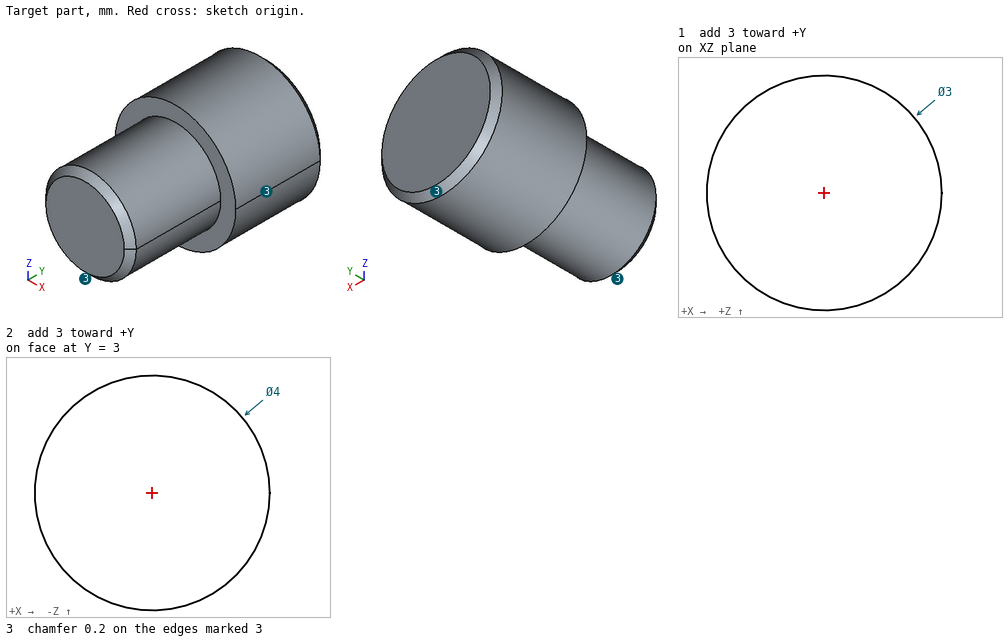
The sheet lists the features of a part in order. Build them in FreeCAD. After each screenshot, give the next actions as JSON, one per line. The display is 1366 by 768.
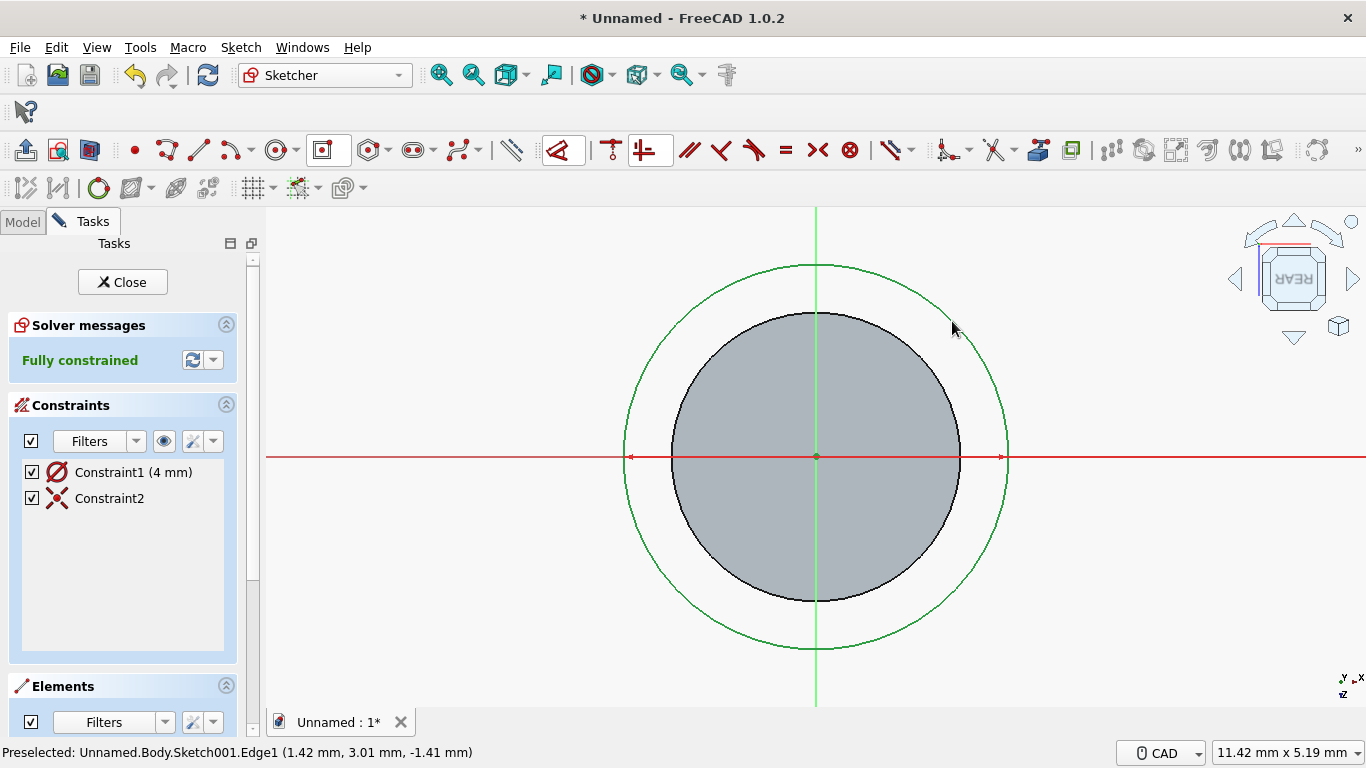
{"action": "left_click", "coordinate": [123, 282]}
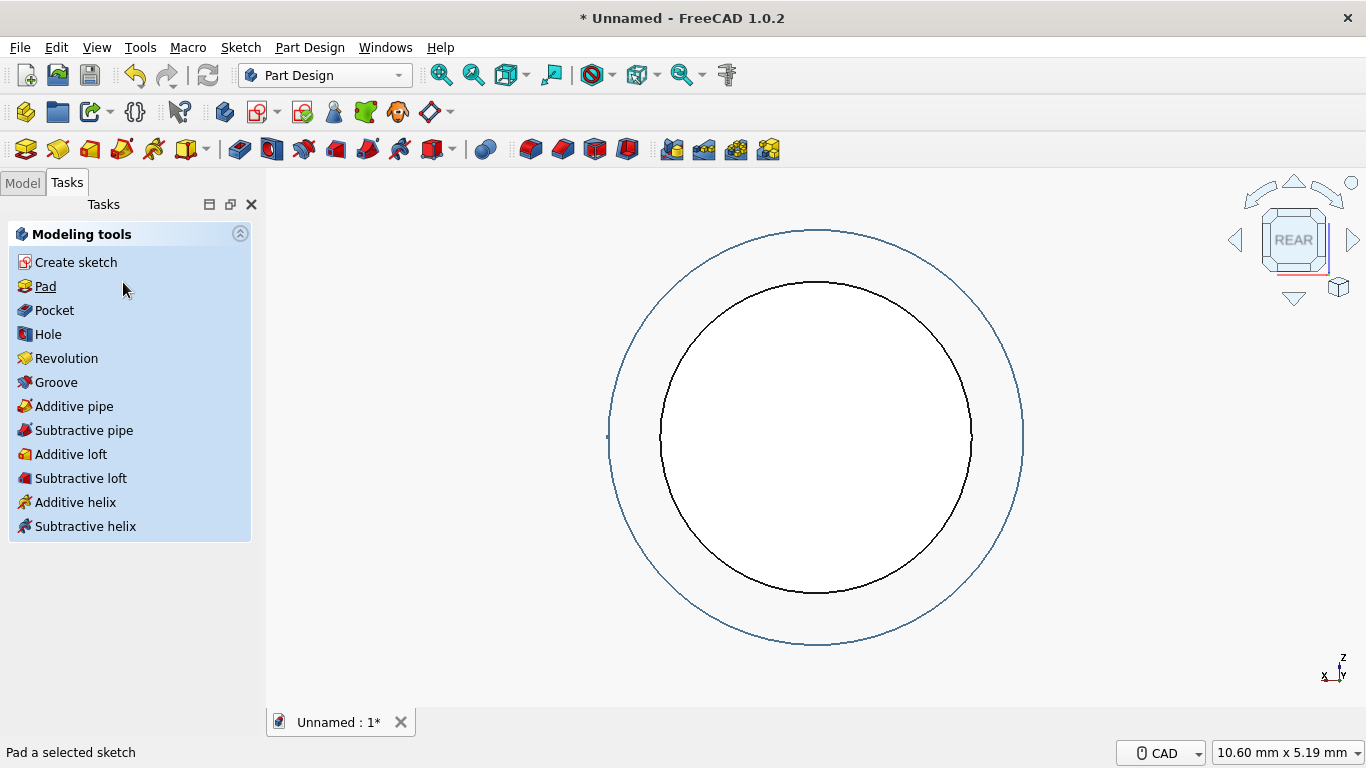
{"action": "left_click", "coordinate": [26, 150]}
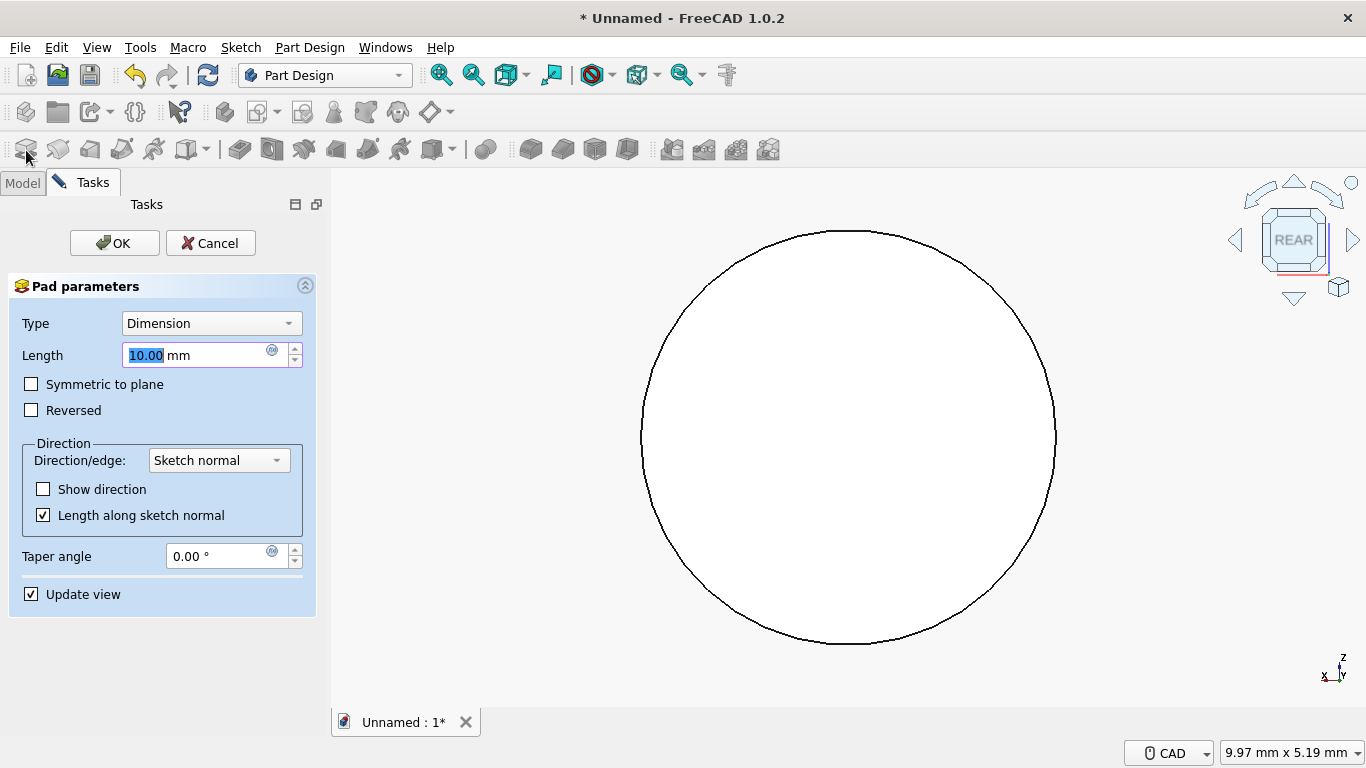
{"action": "type", "text": "3"}
{"action": "key", "text": "Tab"}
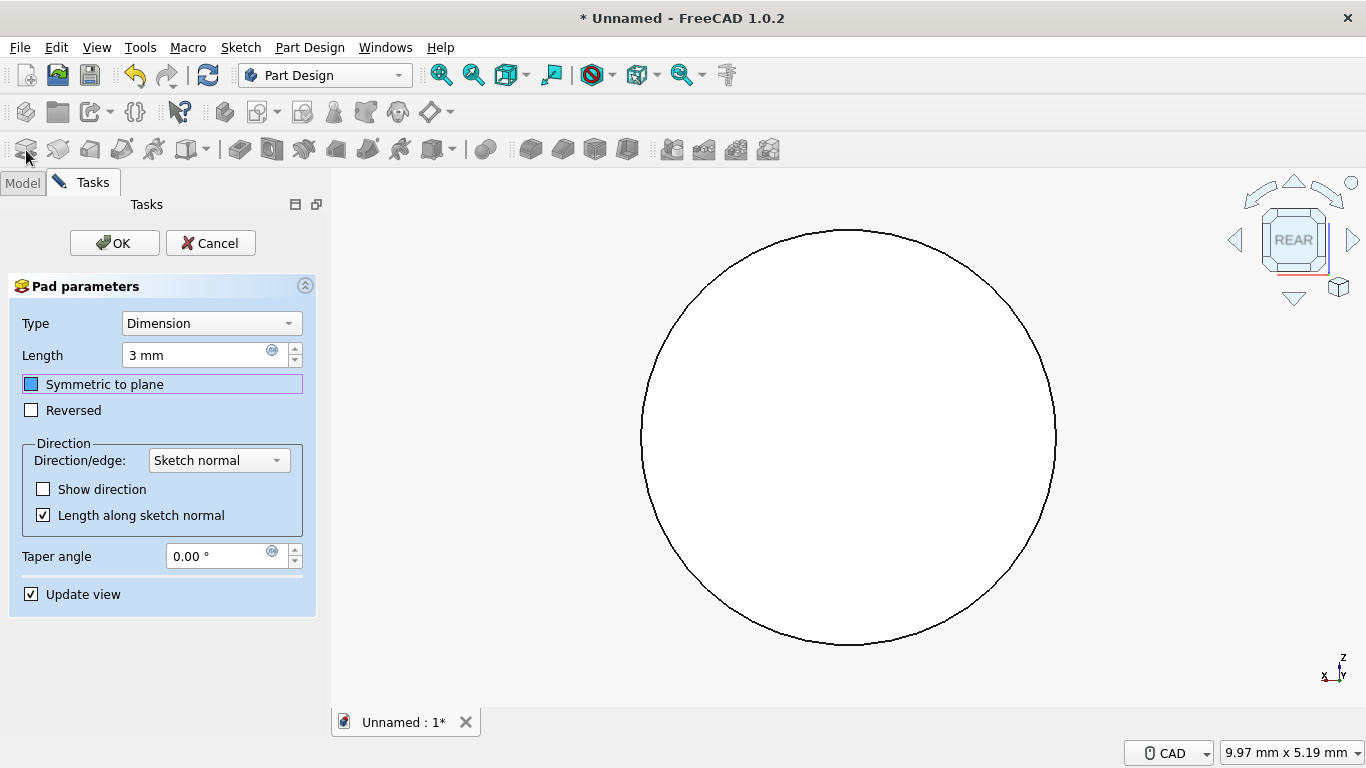
{"action": "left_click", "coordinate": [115, 243]}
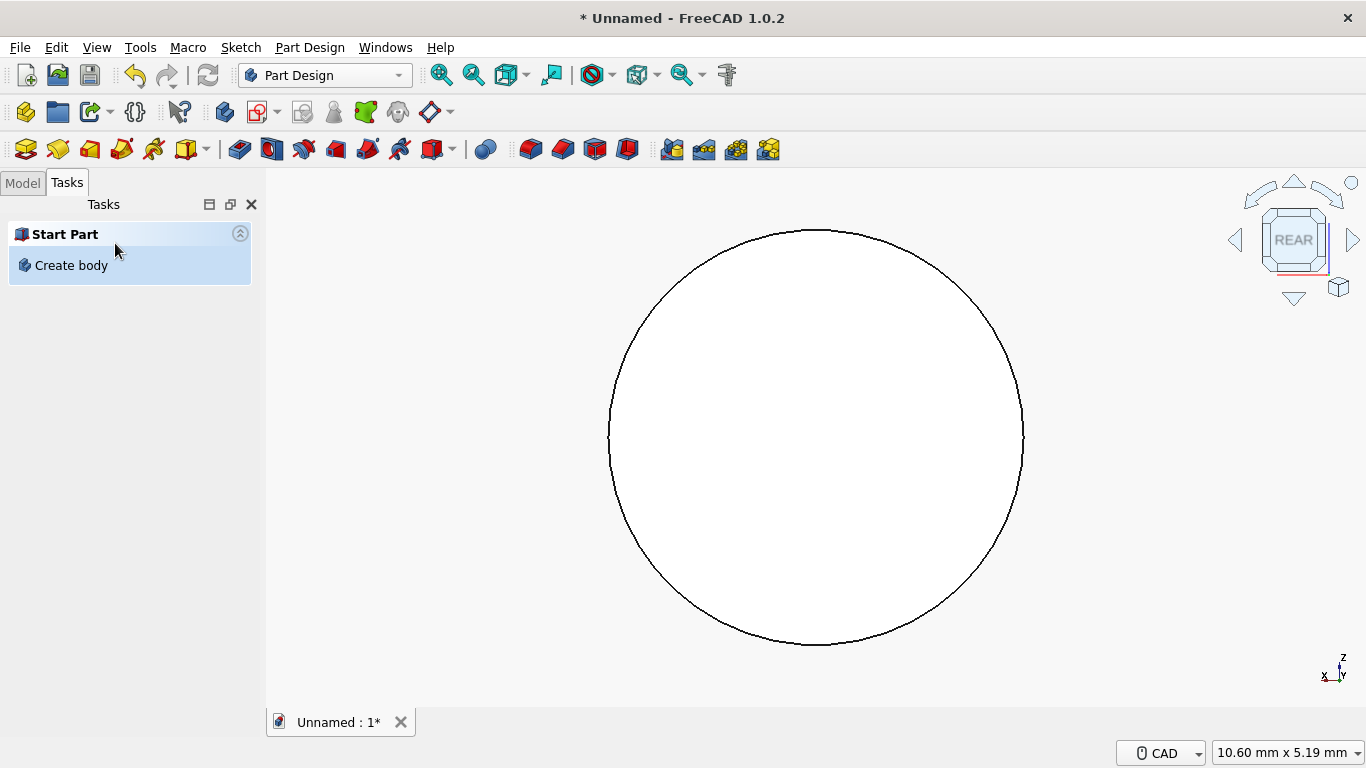
{"action": "left_click", "coordinate": [1024, 436]}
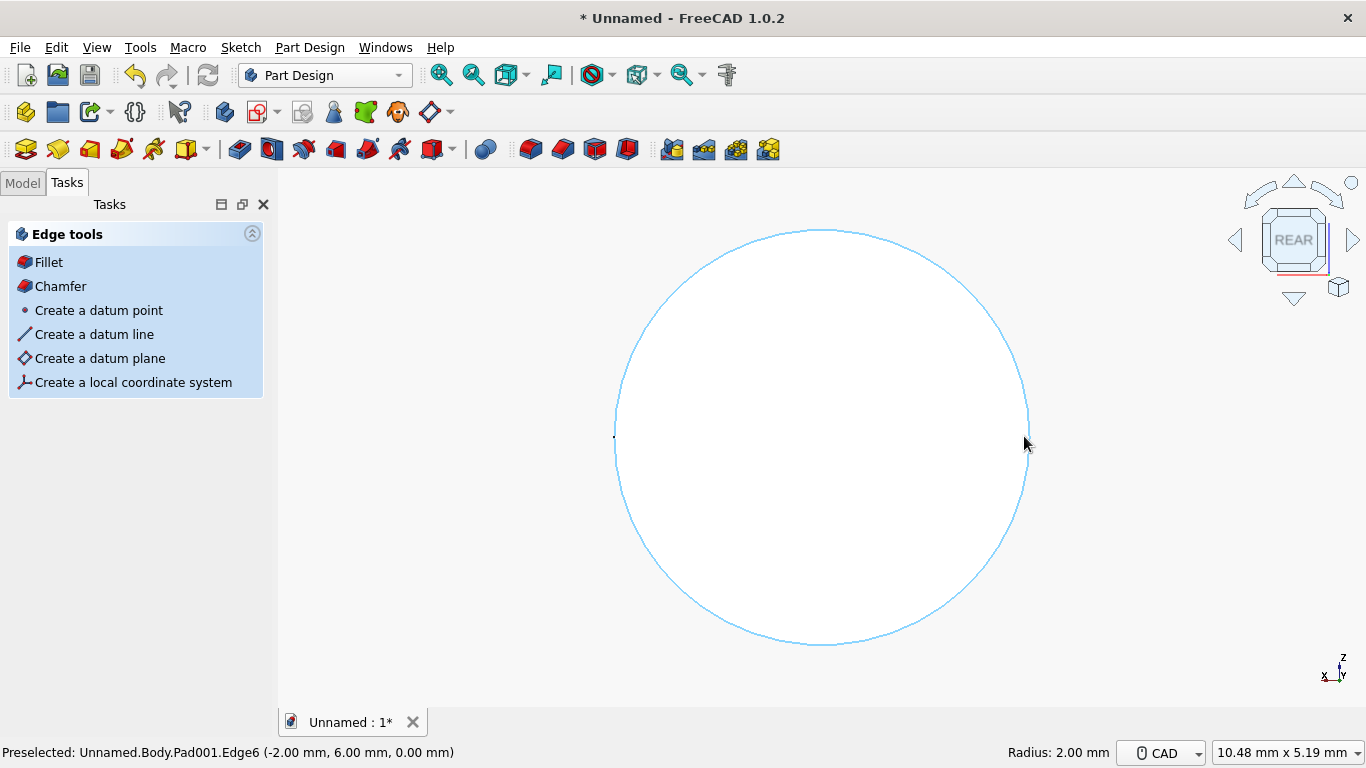
{"action": "key", "text": "0"}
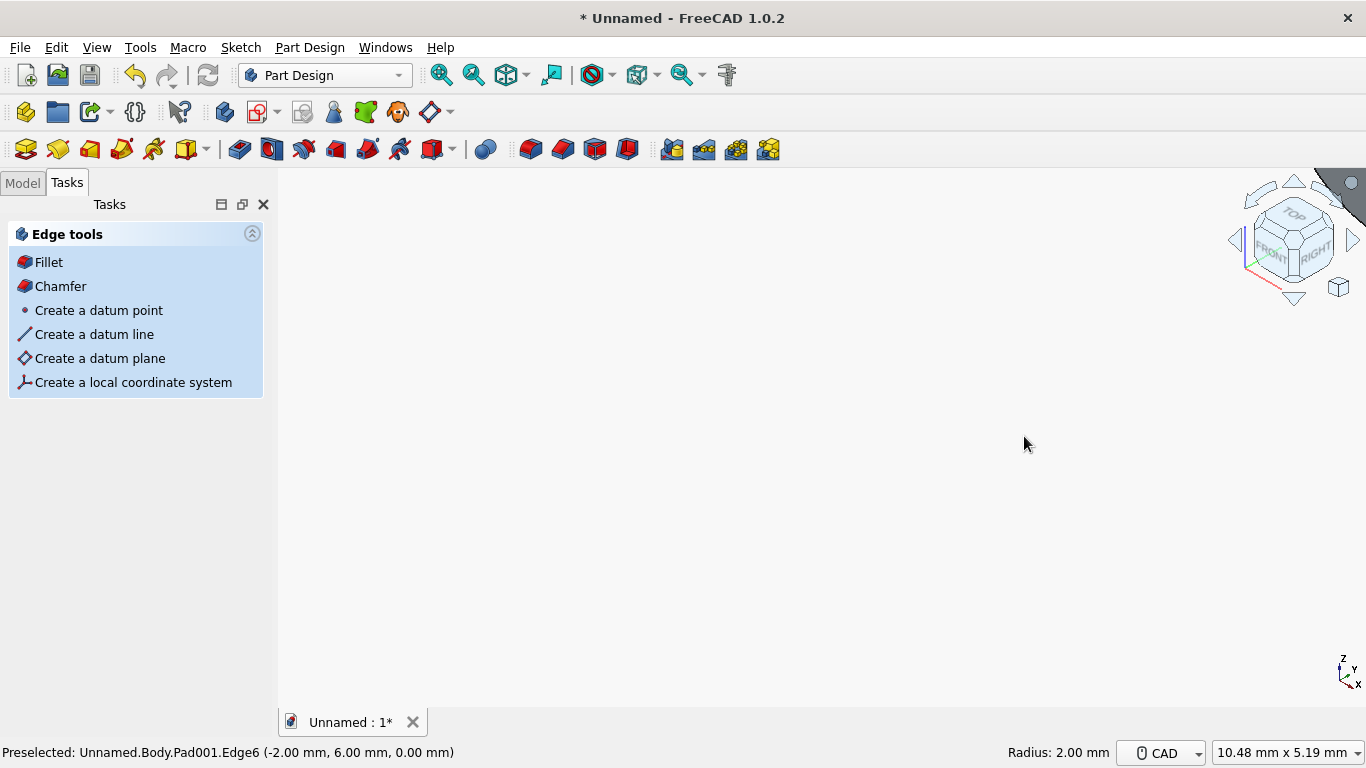
{"action": "key", "text": "v f"}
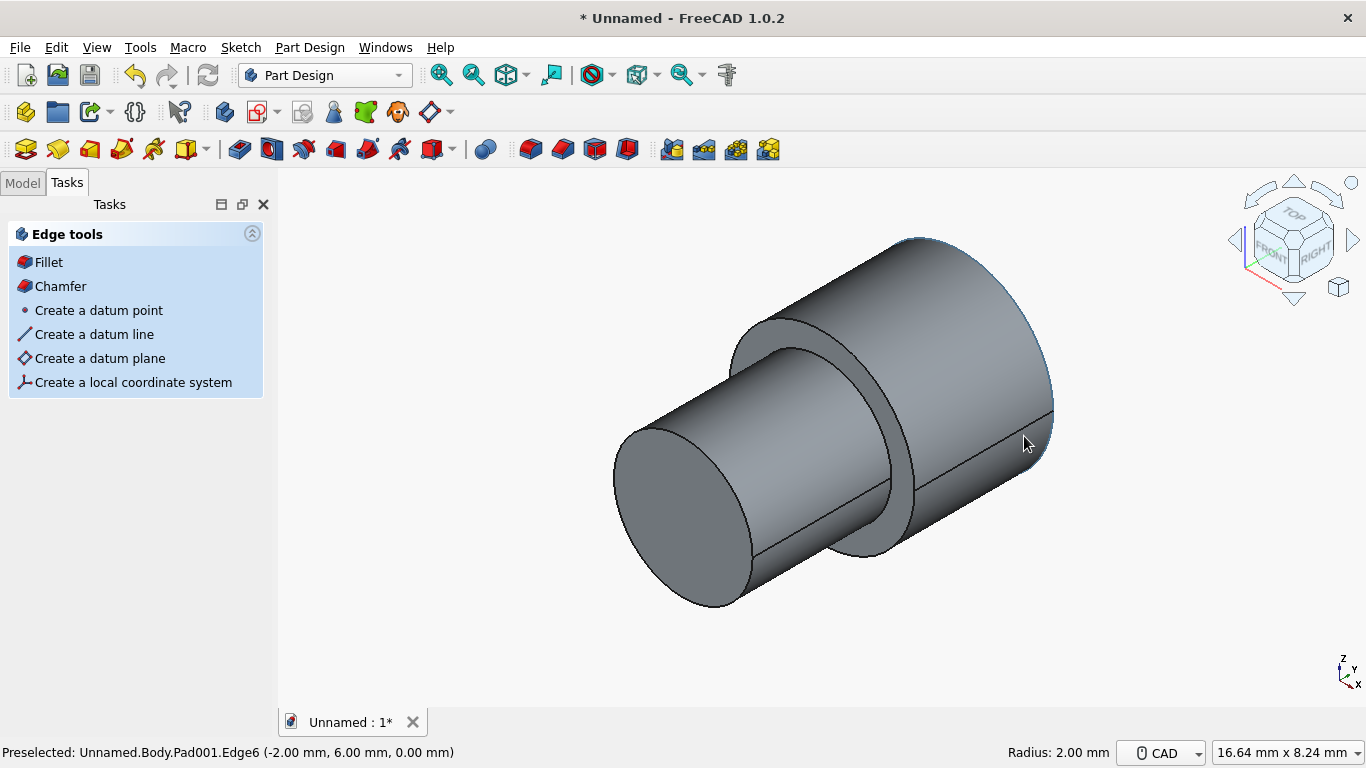
{"action": "left_click", "coordinate": [662, 428], "text": "ctrl"}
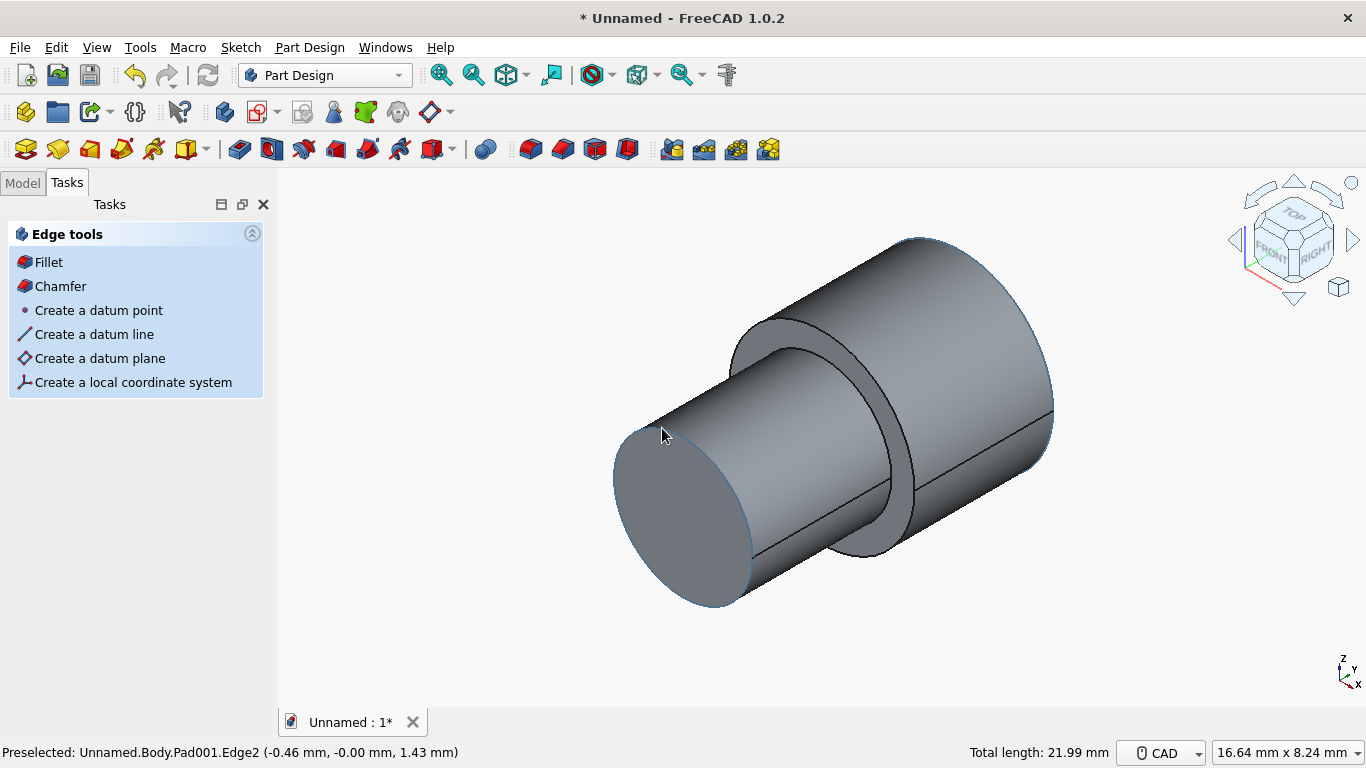
{"action": "left_click", "coordinate": [564, 150]}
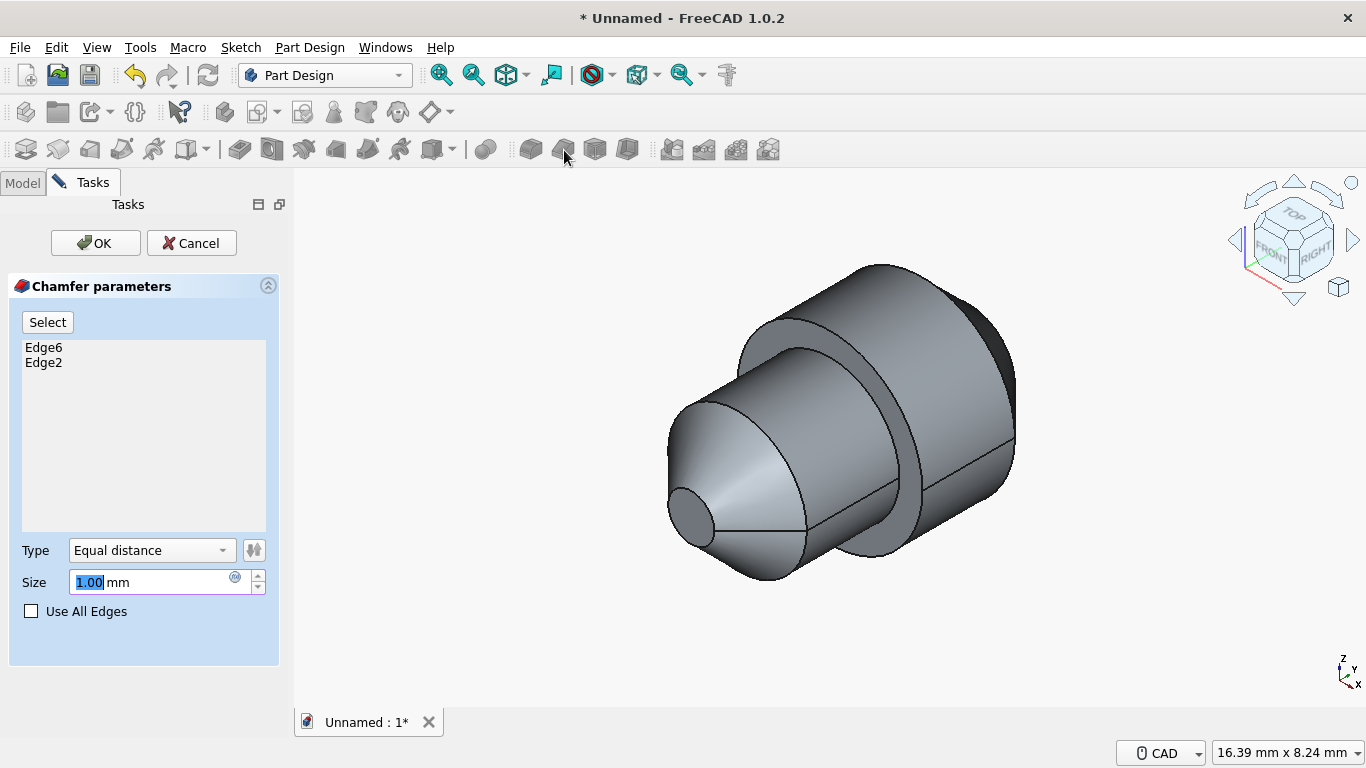
{"action": "type", "text": "0.2"}
{"action": "key", "text": "Tab"}